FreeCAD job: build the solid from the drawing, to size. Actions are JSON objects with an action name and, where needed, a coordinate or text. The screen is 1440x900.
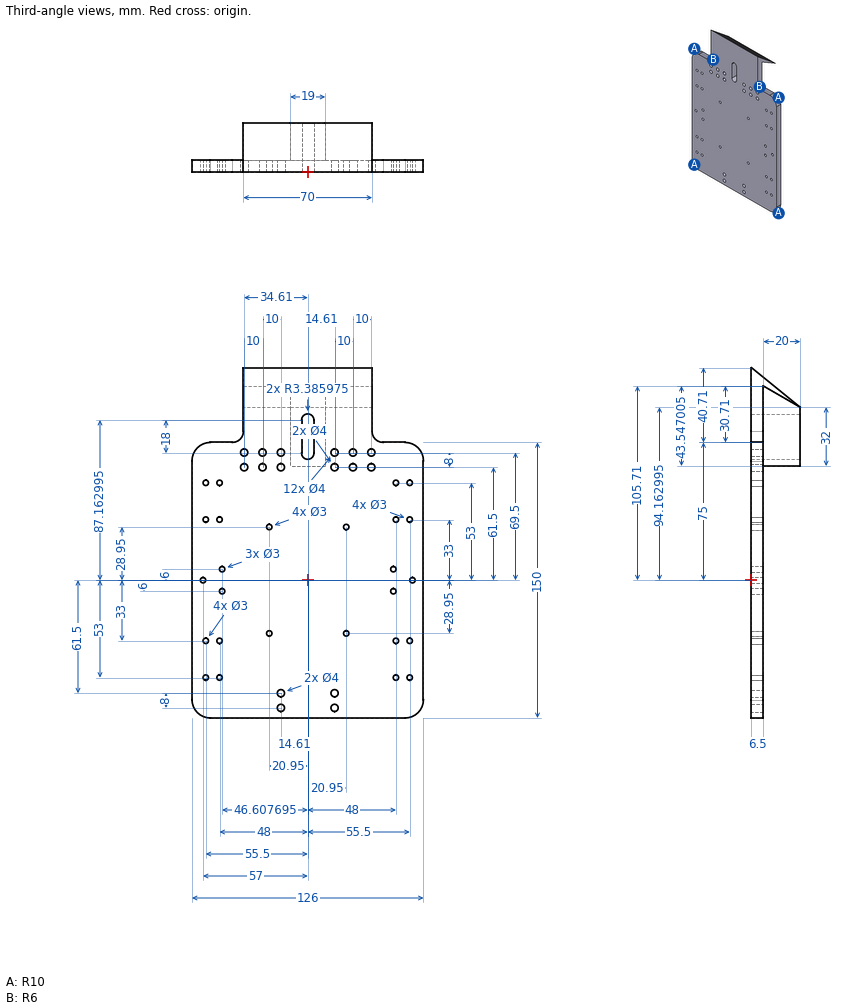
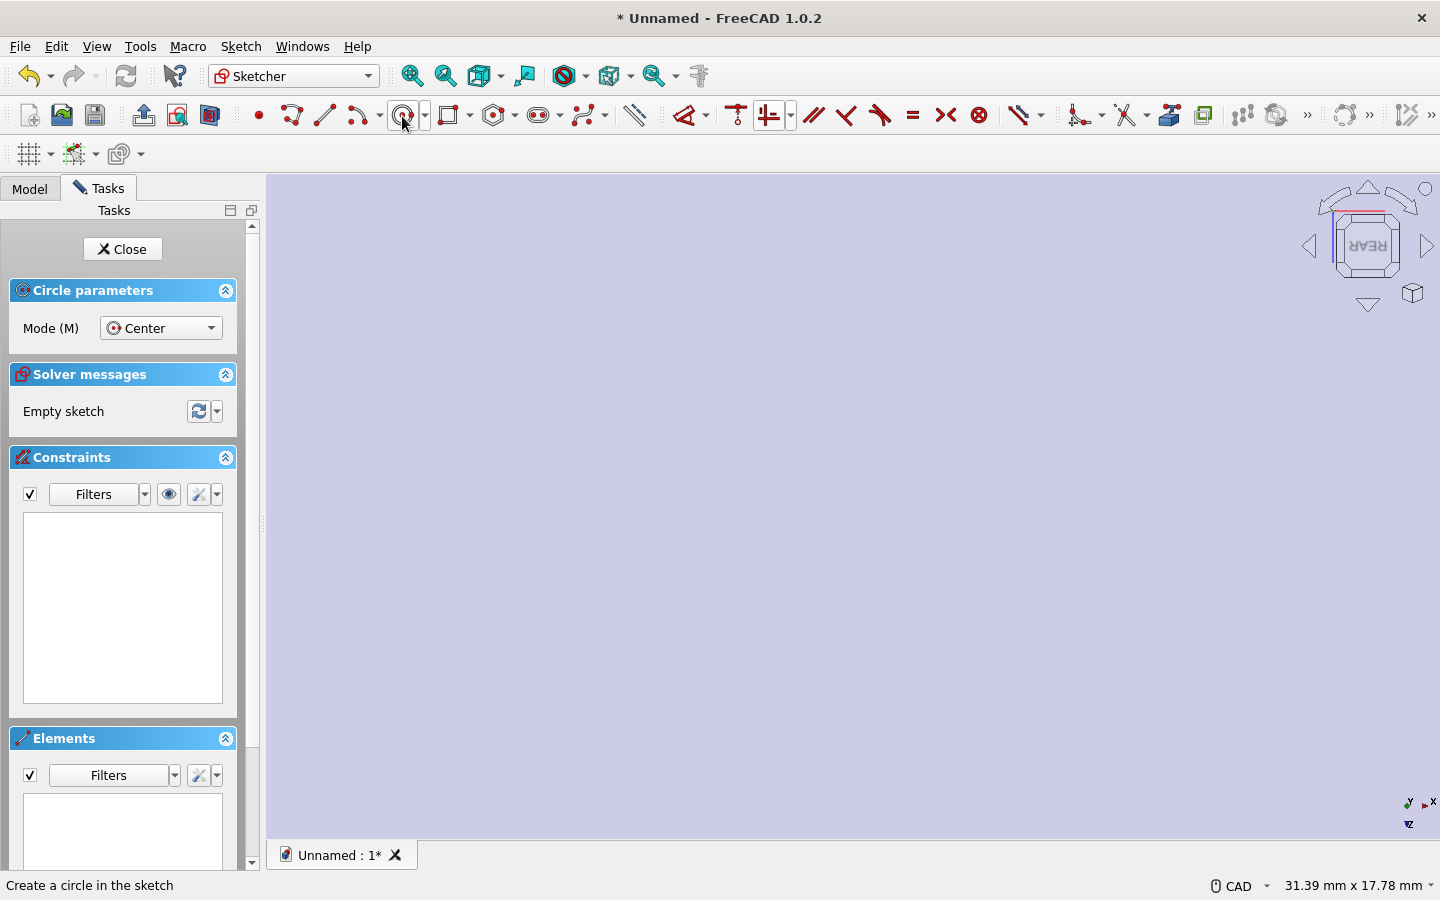
{"action": "left_click", "coordinate": [782, 347]}
{"action": "mouse_move", "coordinate": [835, 294]}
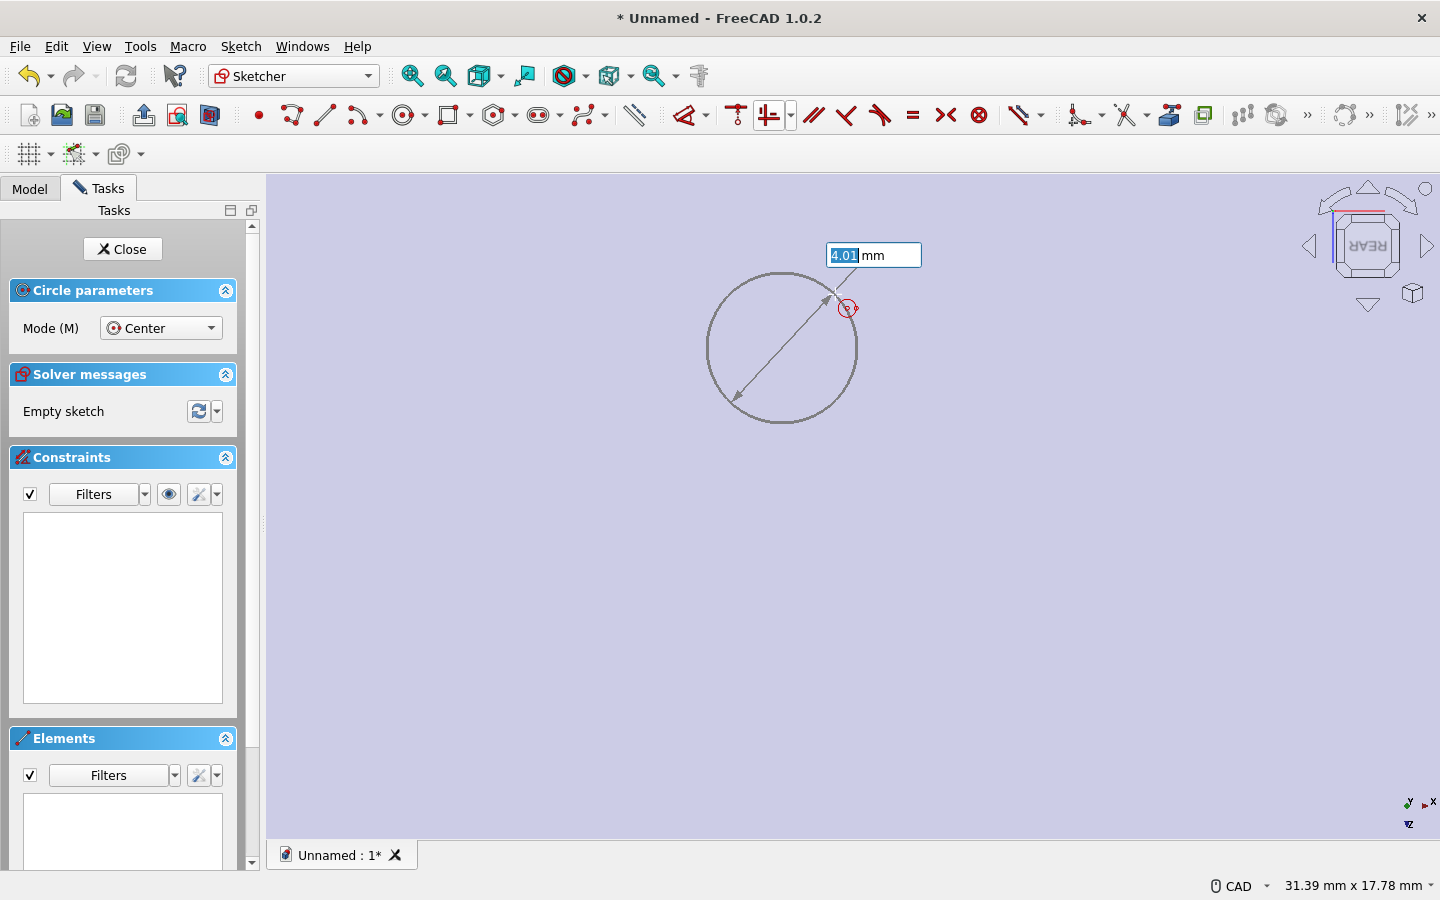
{"action": "type", "text": "4"}
{"action": "key", "text": "Return"}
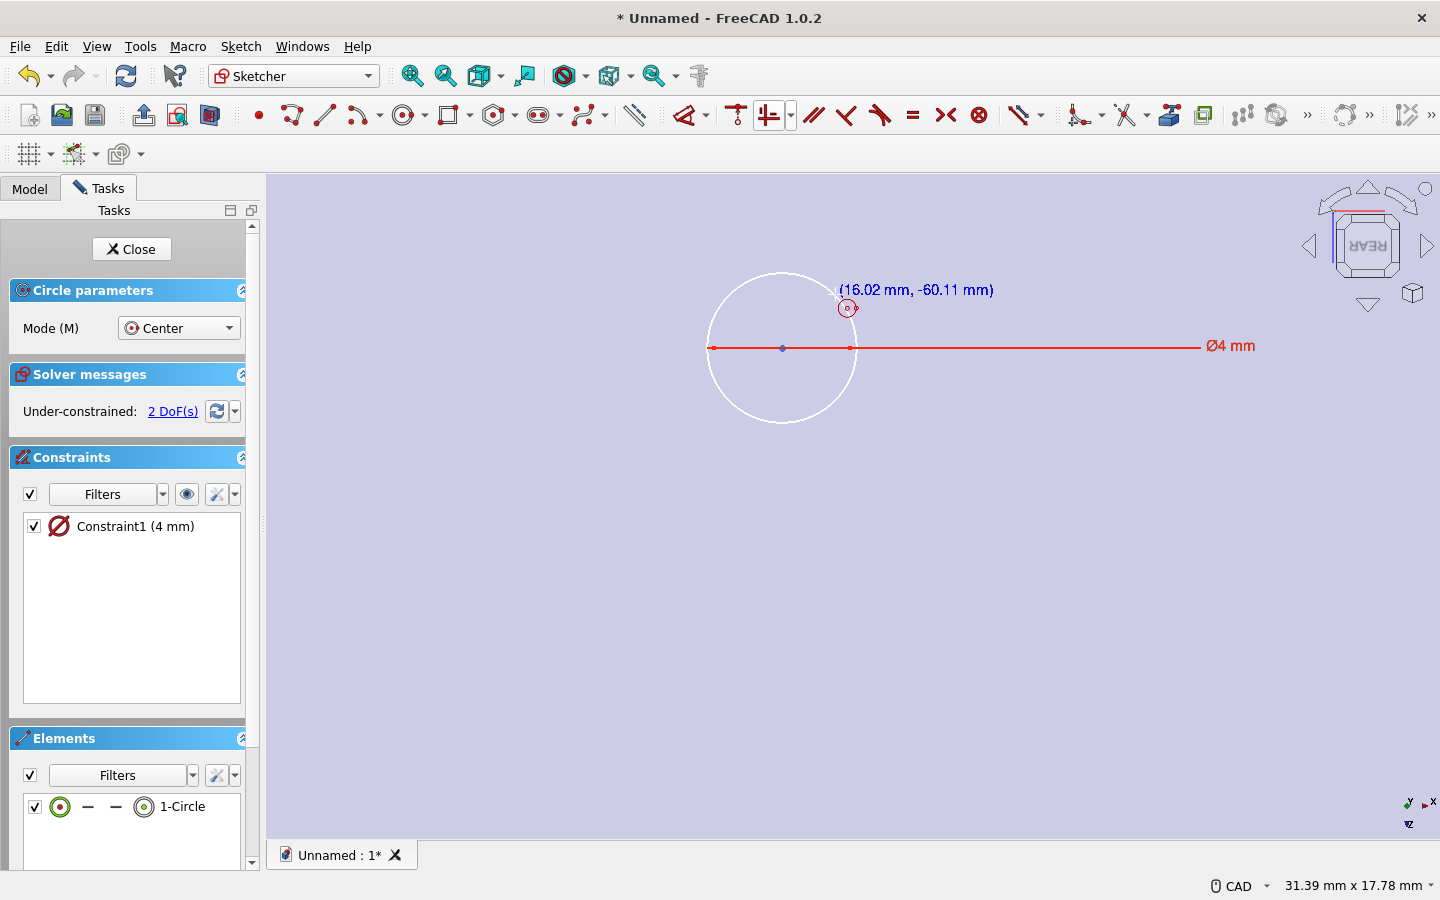
{"action": "left_click", "coordinate": [782, 646]}
{"action": "mouse_move", "coordinate": [835, 593]}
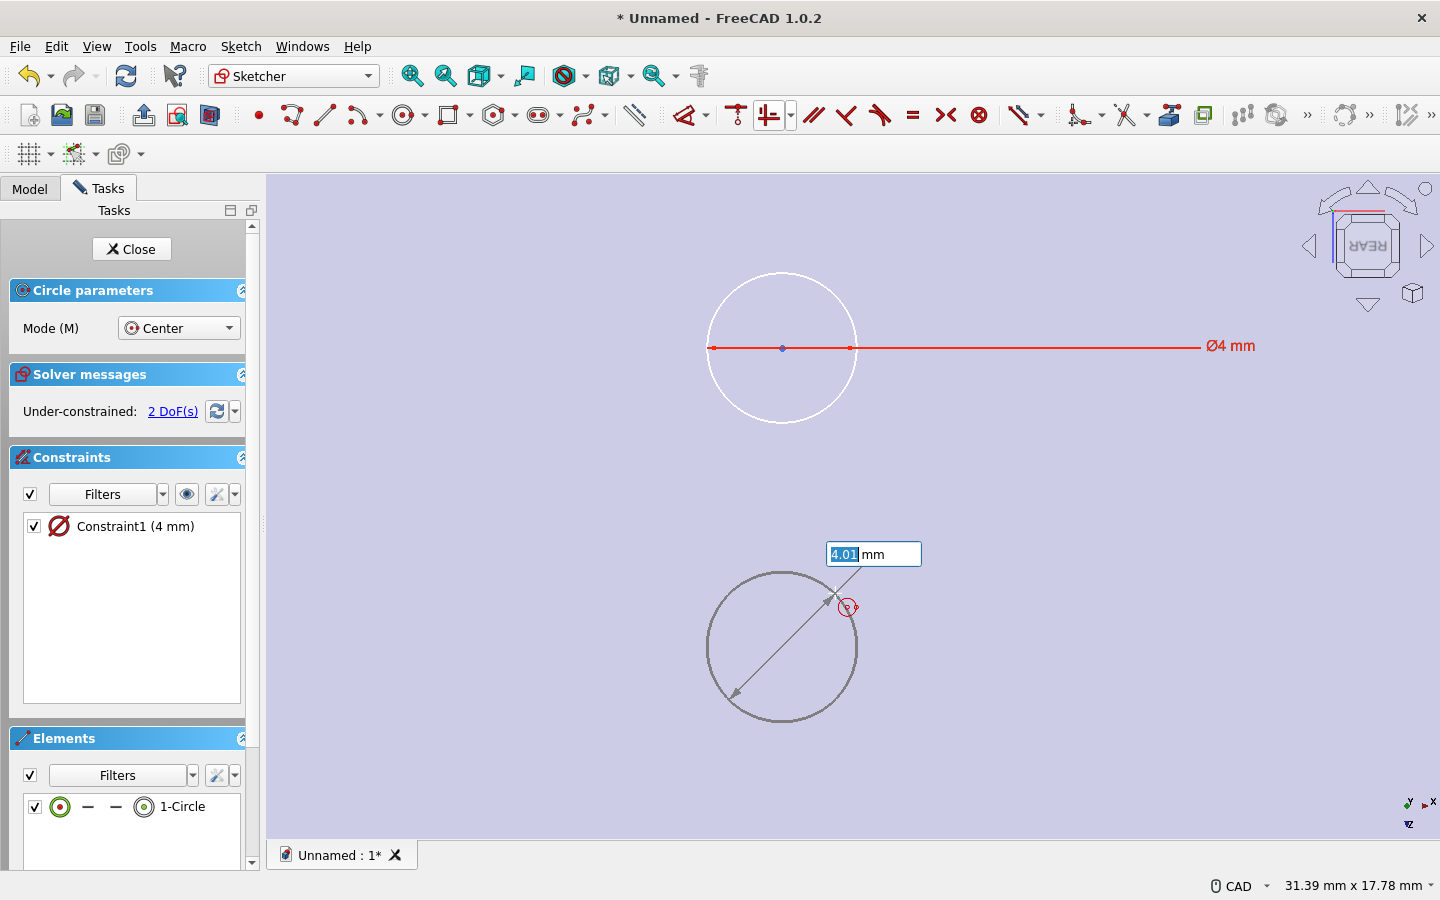
{"action": "type", "text": "4"}
{"action": "key", "text": "Return"}
{"action": "key", "text": "Escape"}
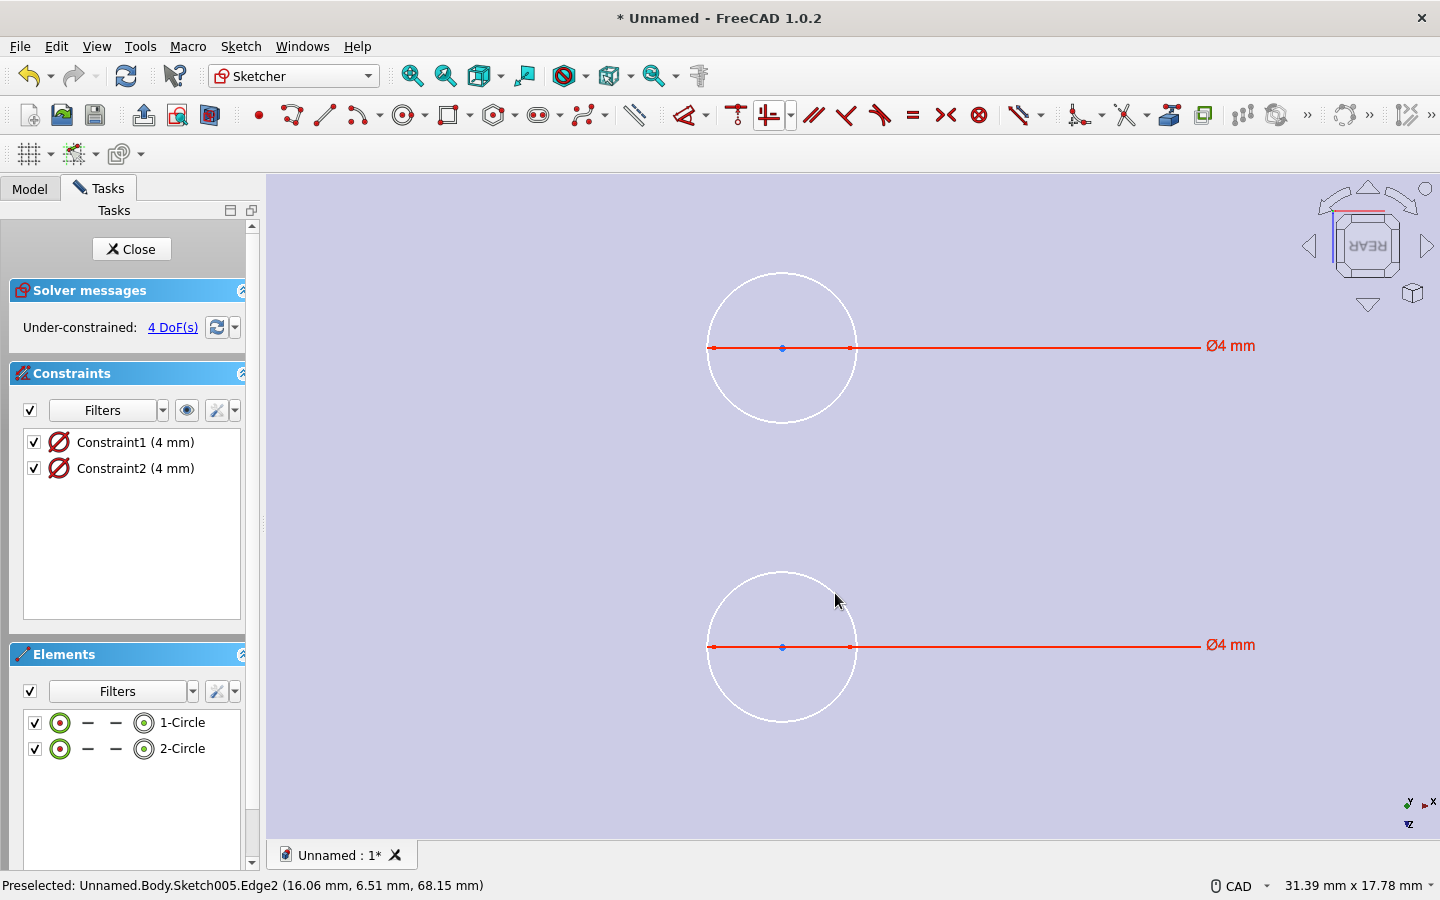
{"action": "left_click", "coordinate": [782, 348]}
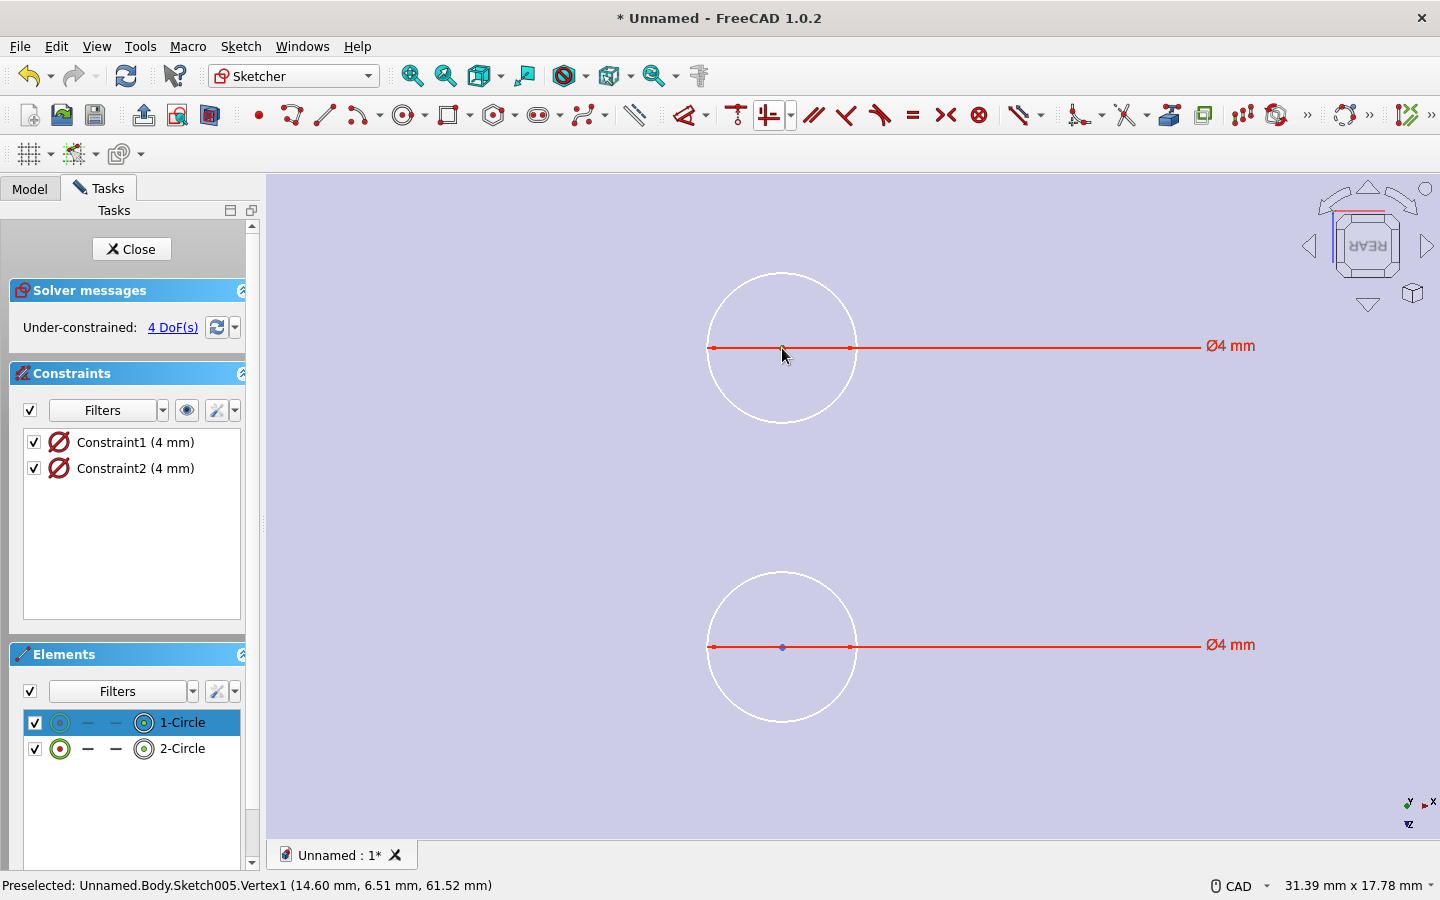
{"action": "left_click", "coordinate": [782, 647]}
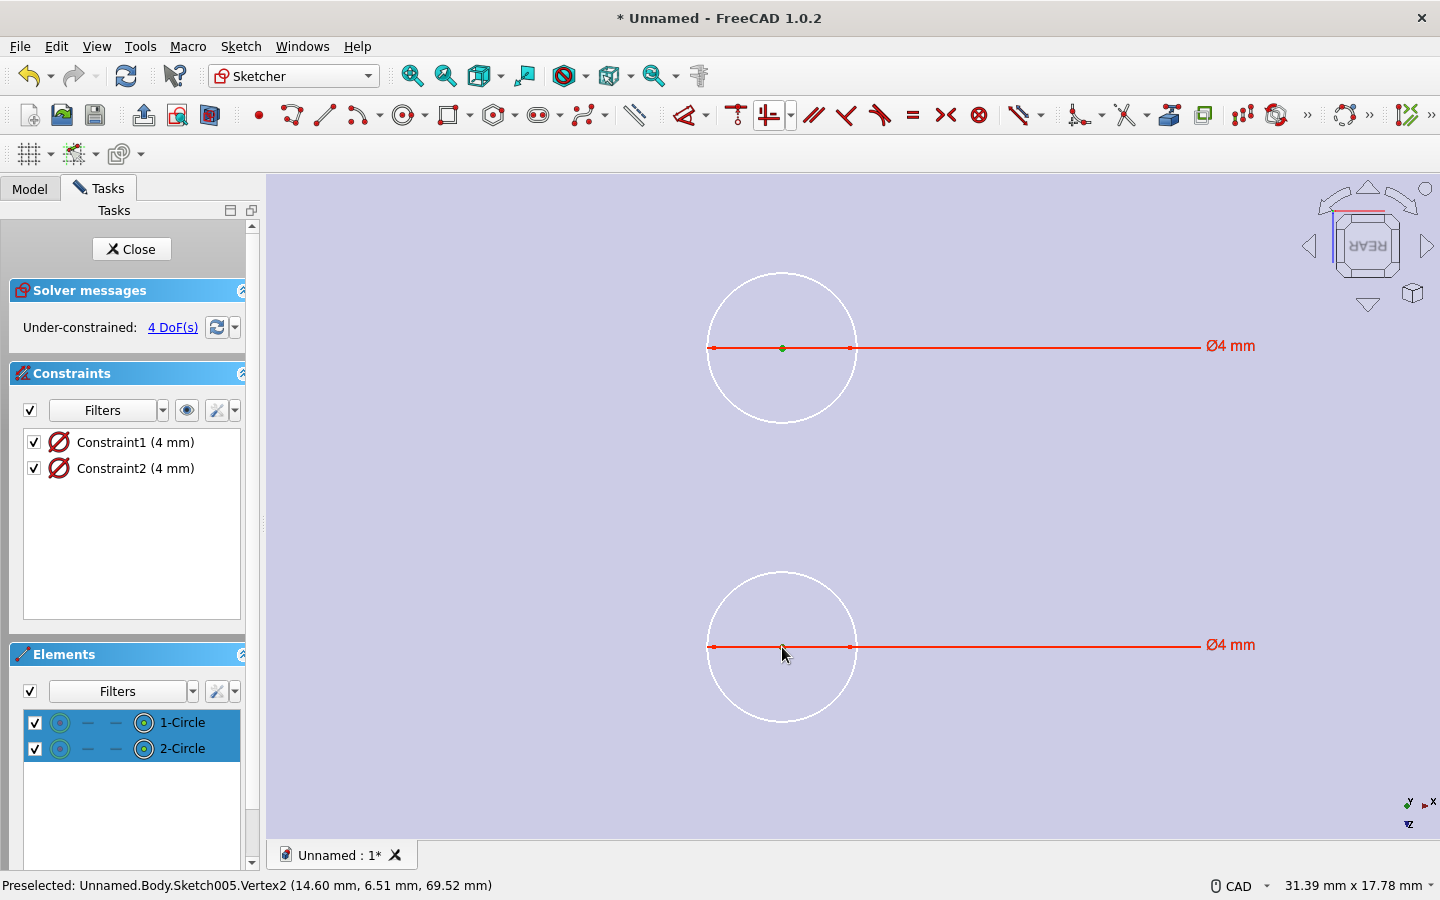
{"action": "key", "text": "v"}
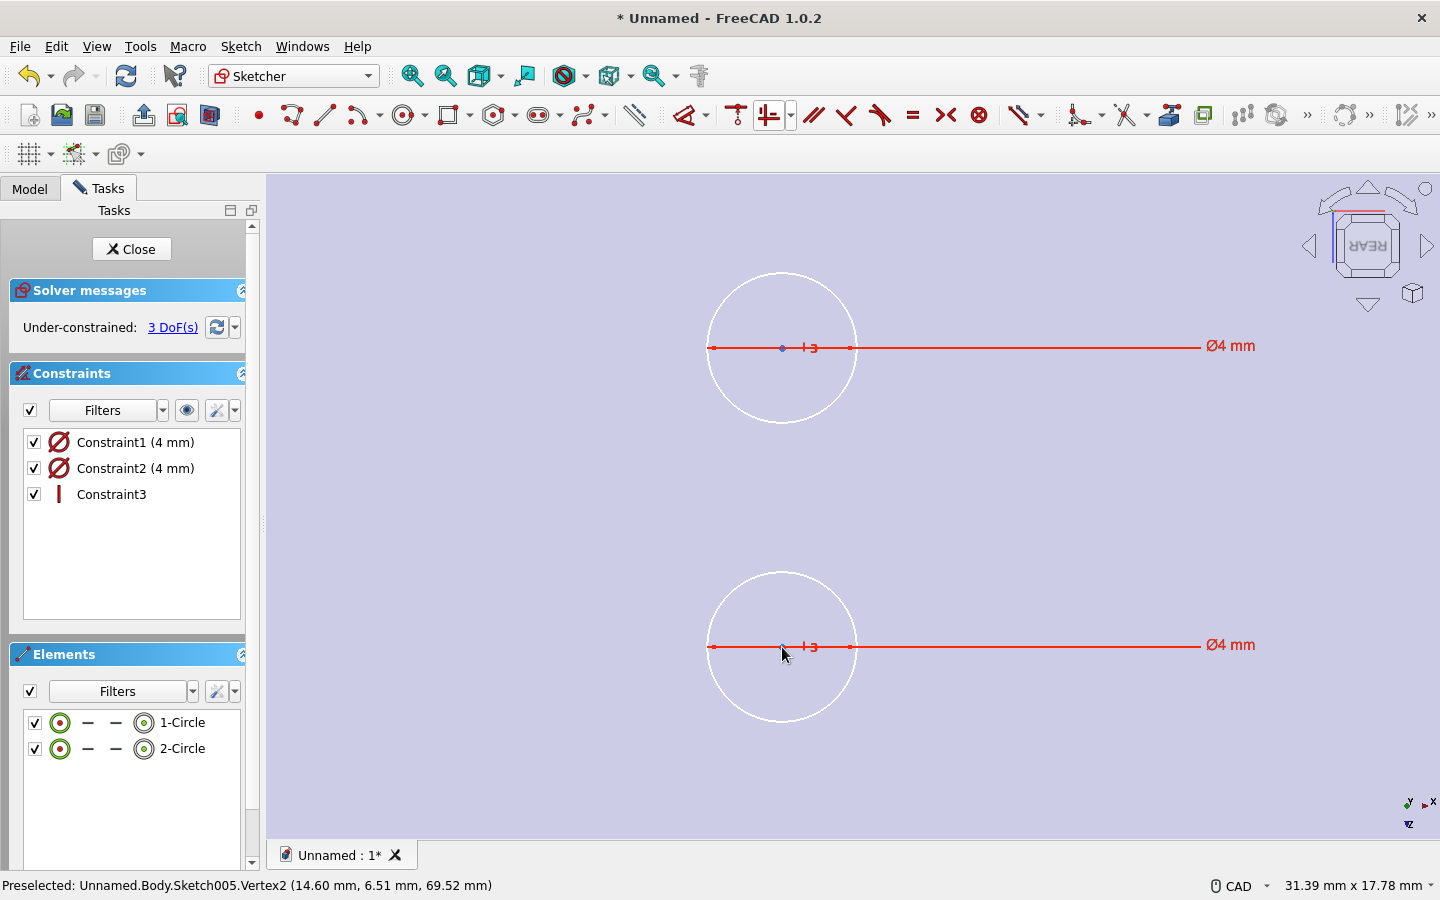
{"action": "left_click", "coordinate": [684, 116]}